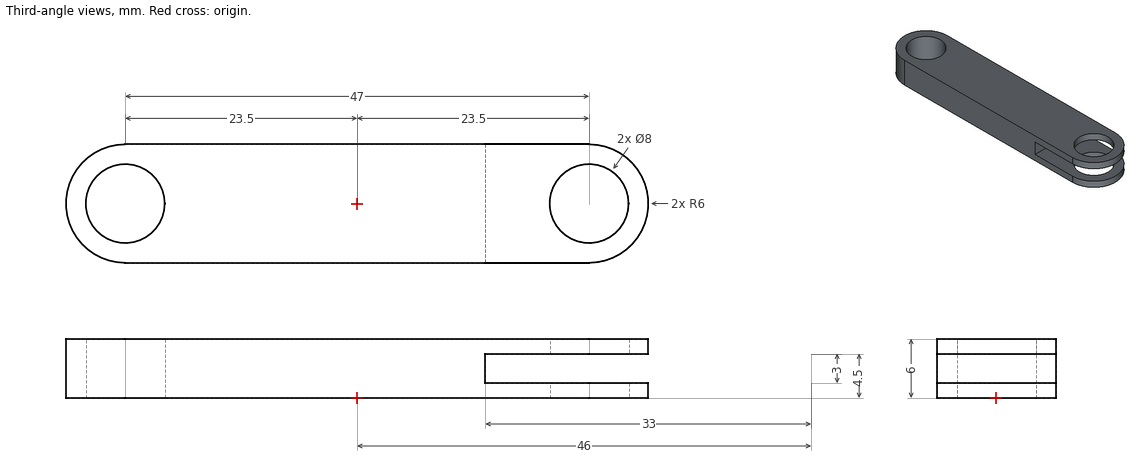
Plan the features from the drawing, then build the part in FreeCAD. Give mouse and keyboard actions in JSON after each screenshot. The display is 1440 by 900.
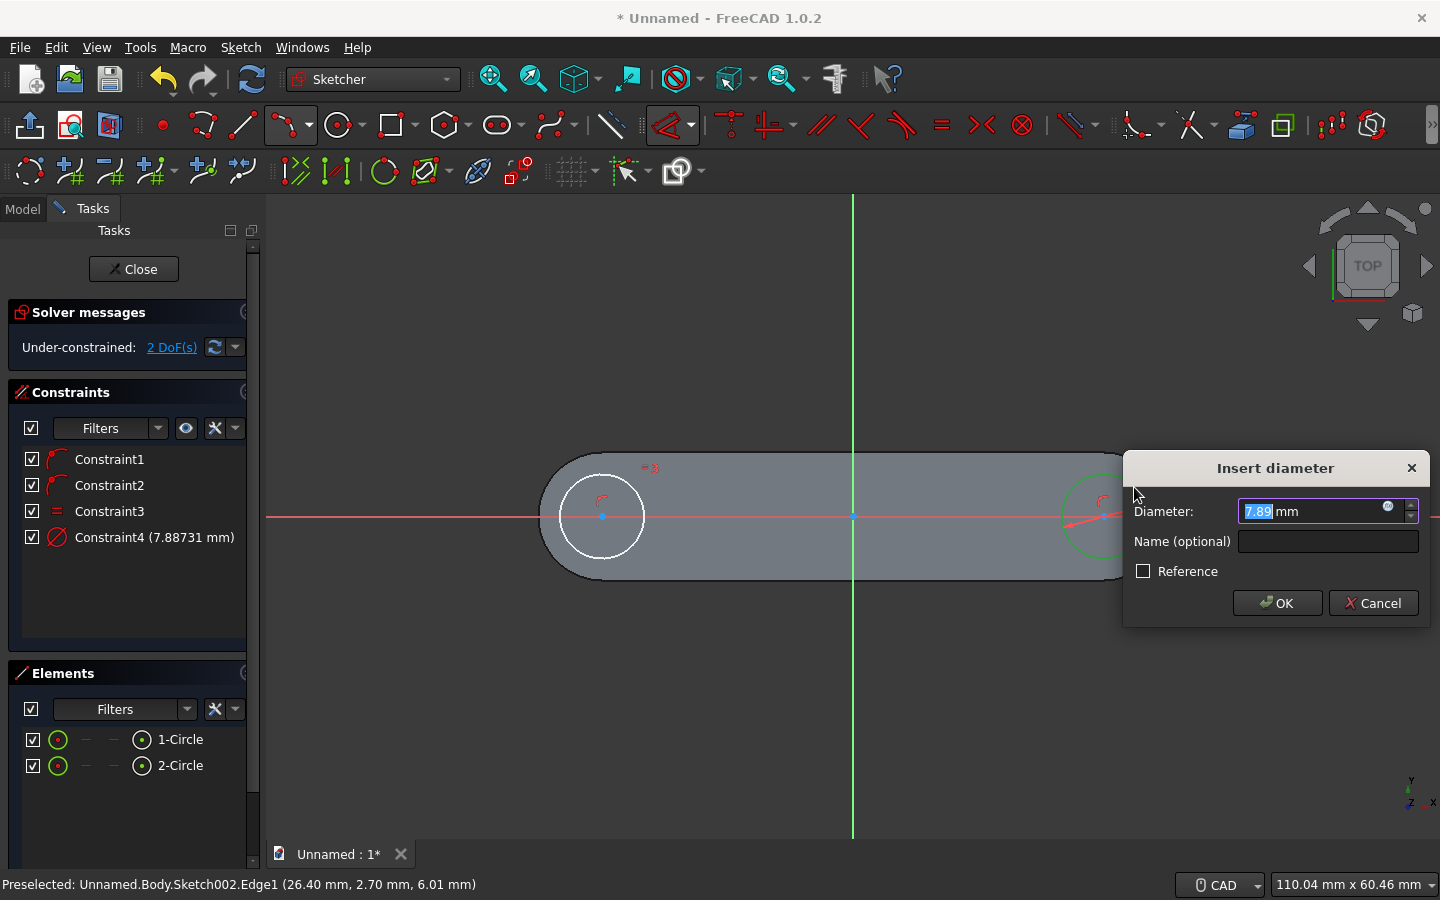
{"action": "type", "text": "8"}
{"action": "key", "text": "Return"}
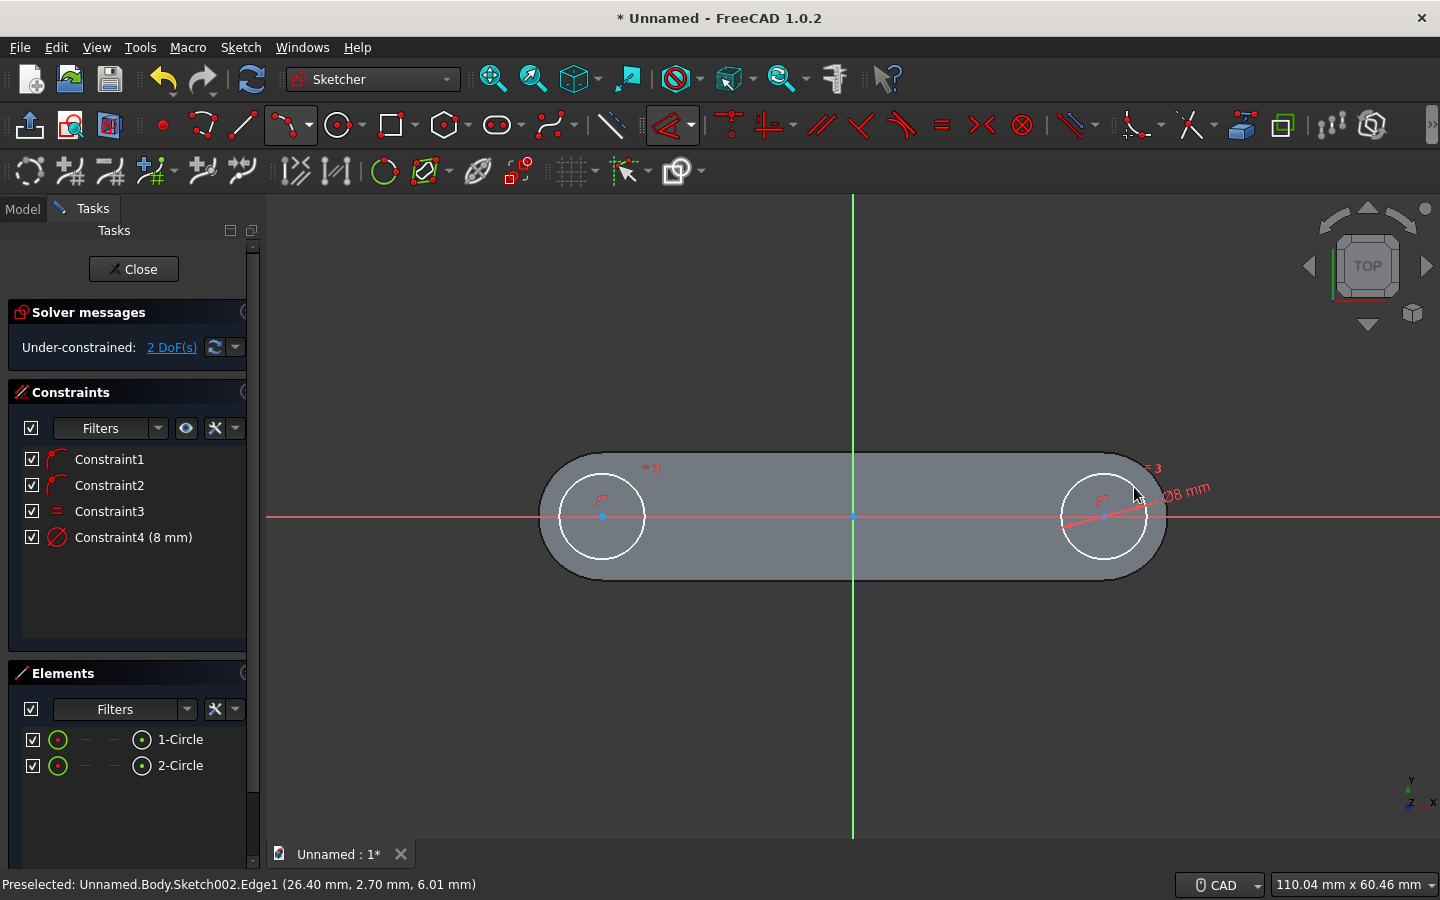
{"action": "left_click", "coordinate": [1104, 516]}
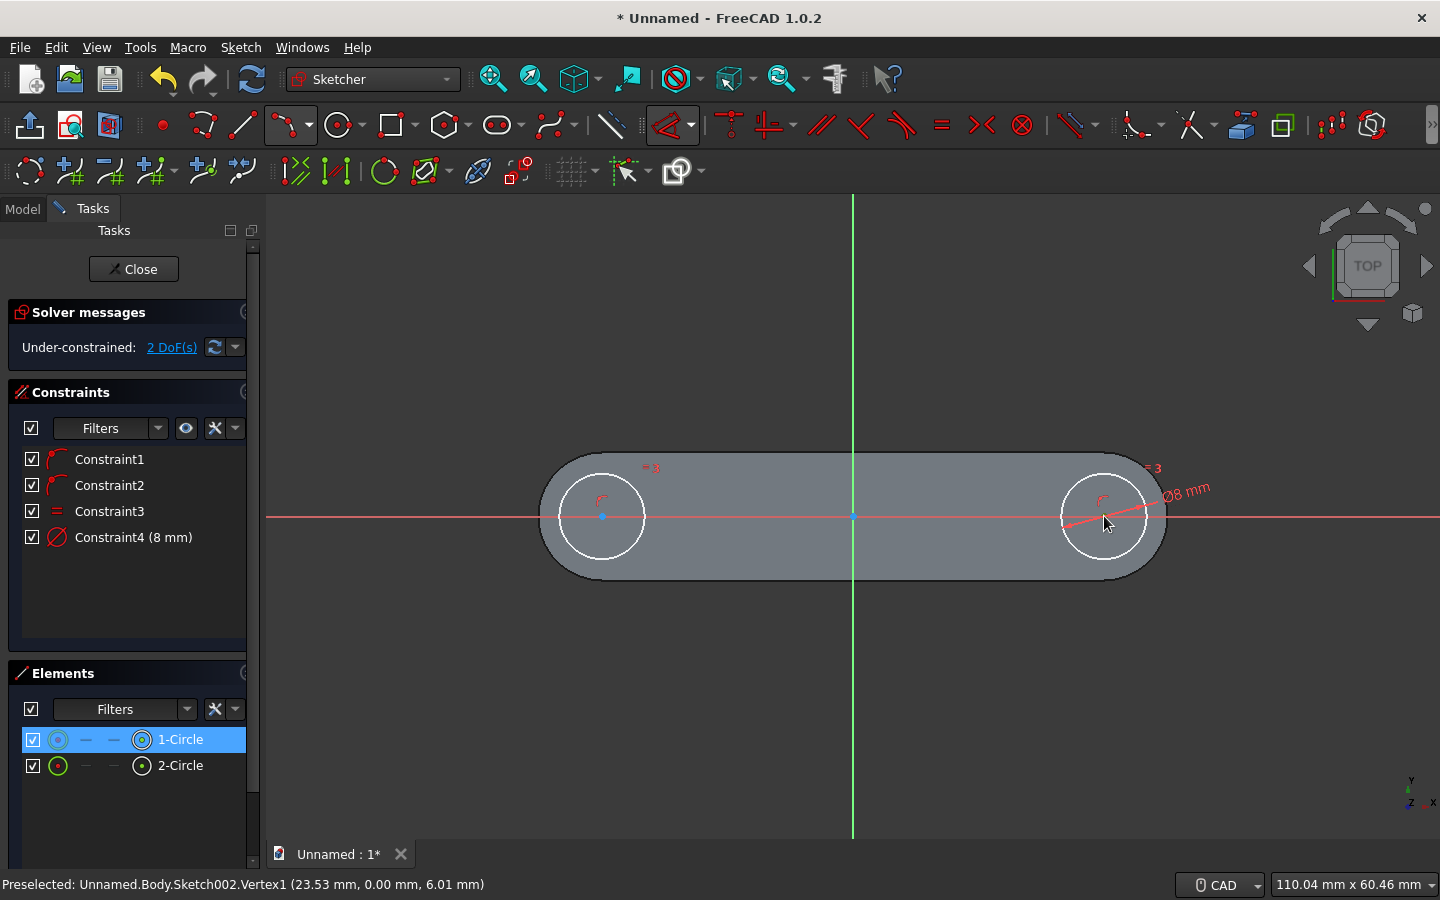
{"action": "left_click", "coordinate": [602, 516]}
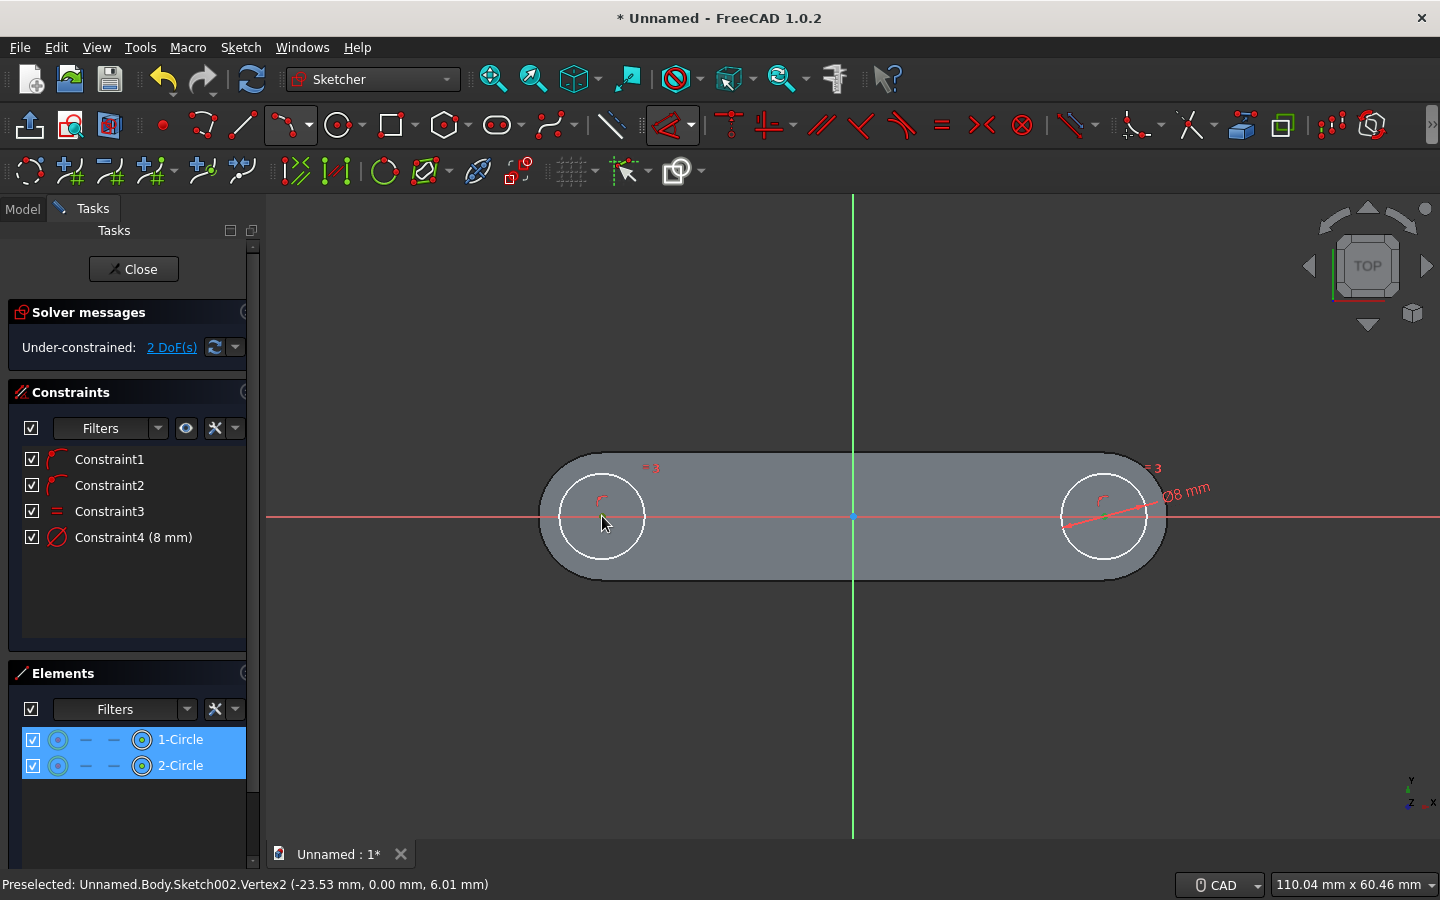
{"action": "key", "text": "l"}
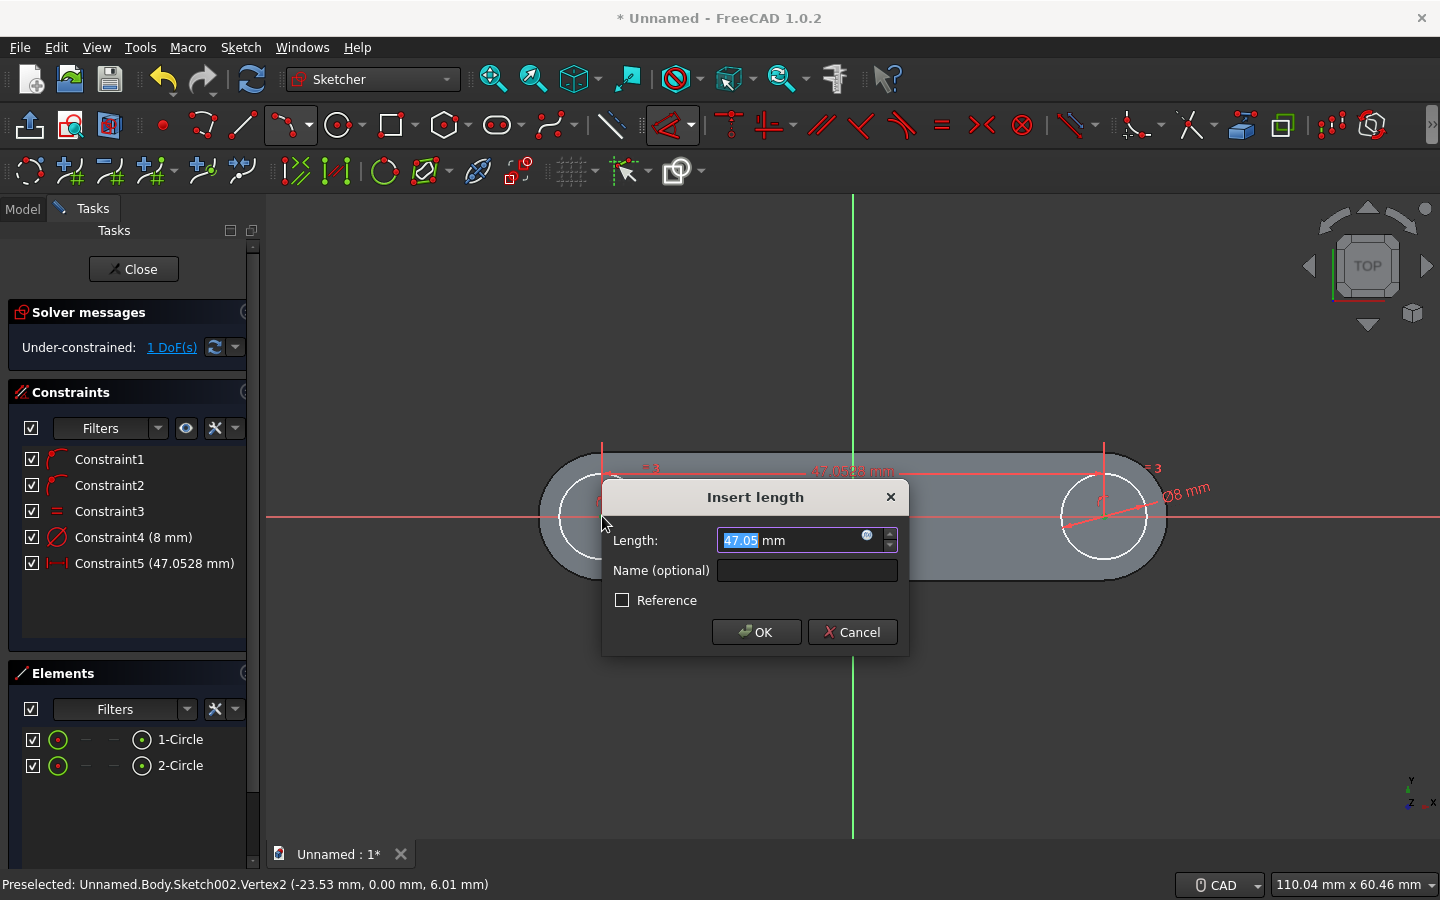
{"action": "type", "text": "47"}
{"action": "key", "text": "Return"}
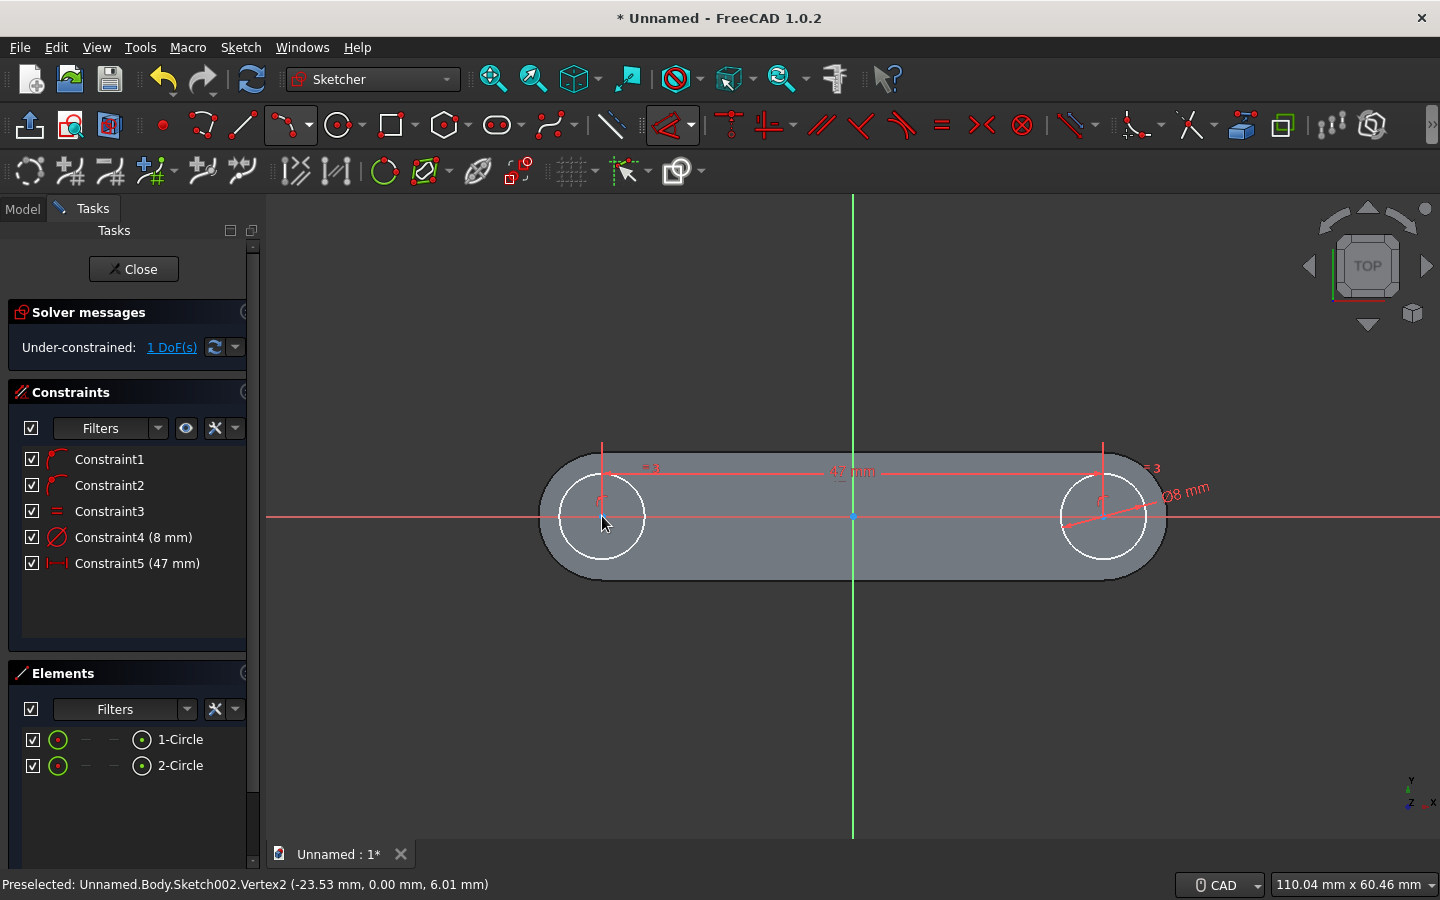
{"action": "left_click", "coordinate": [1103, 516]}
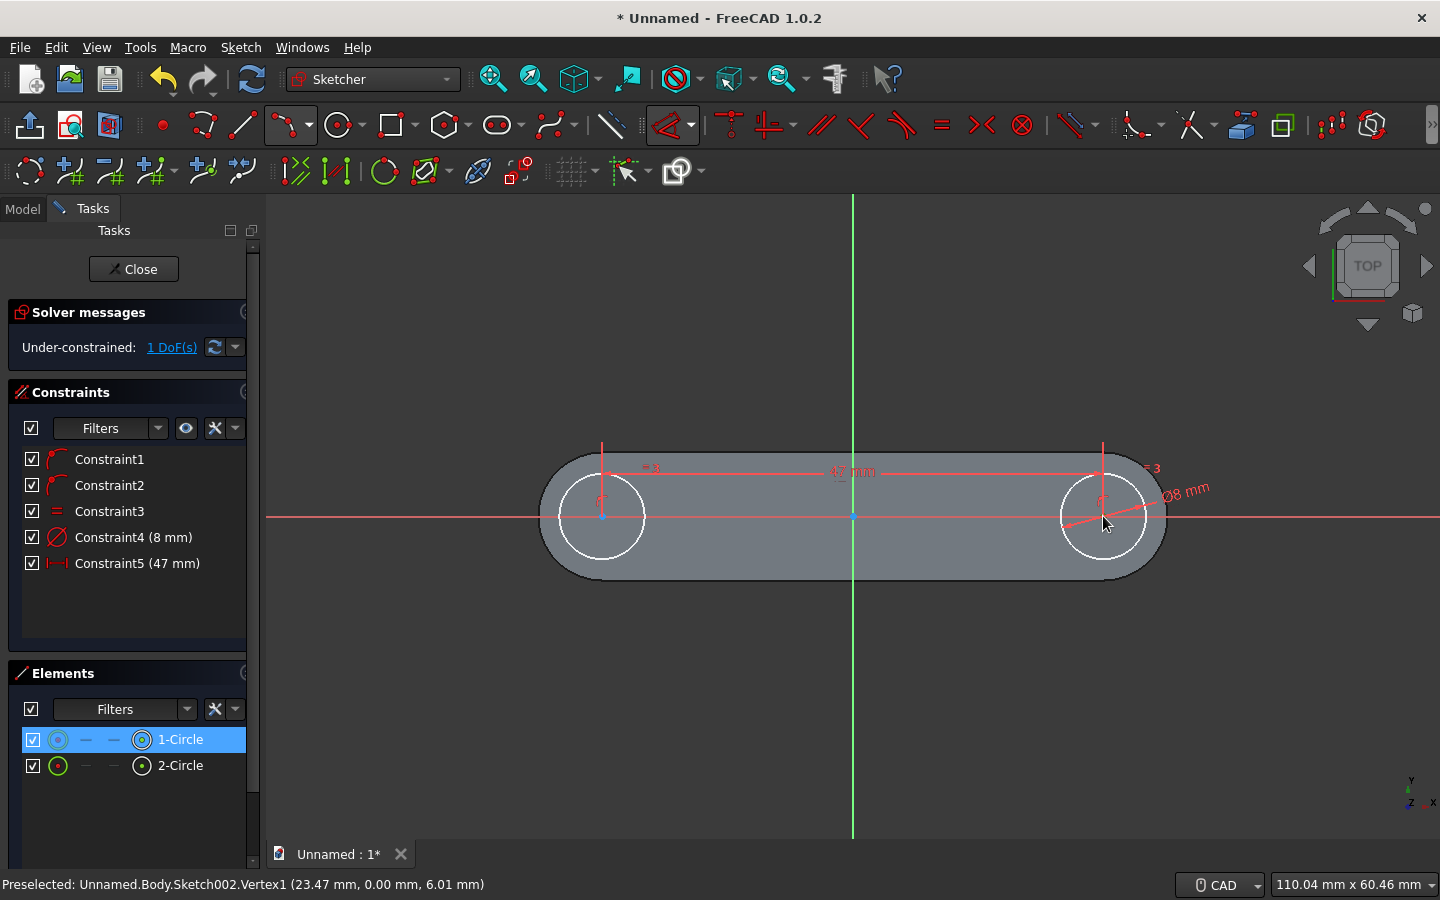
{"action": "key", "text": "l"}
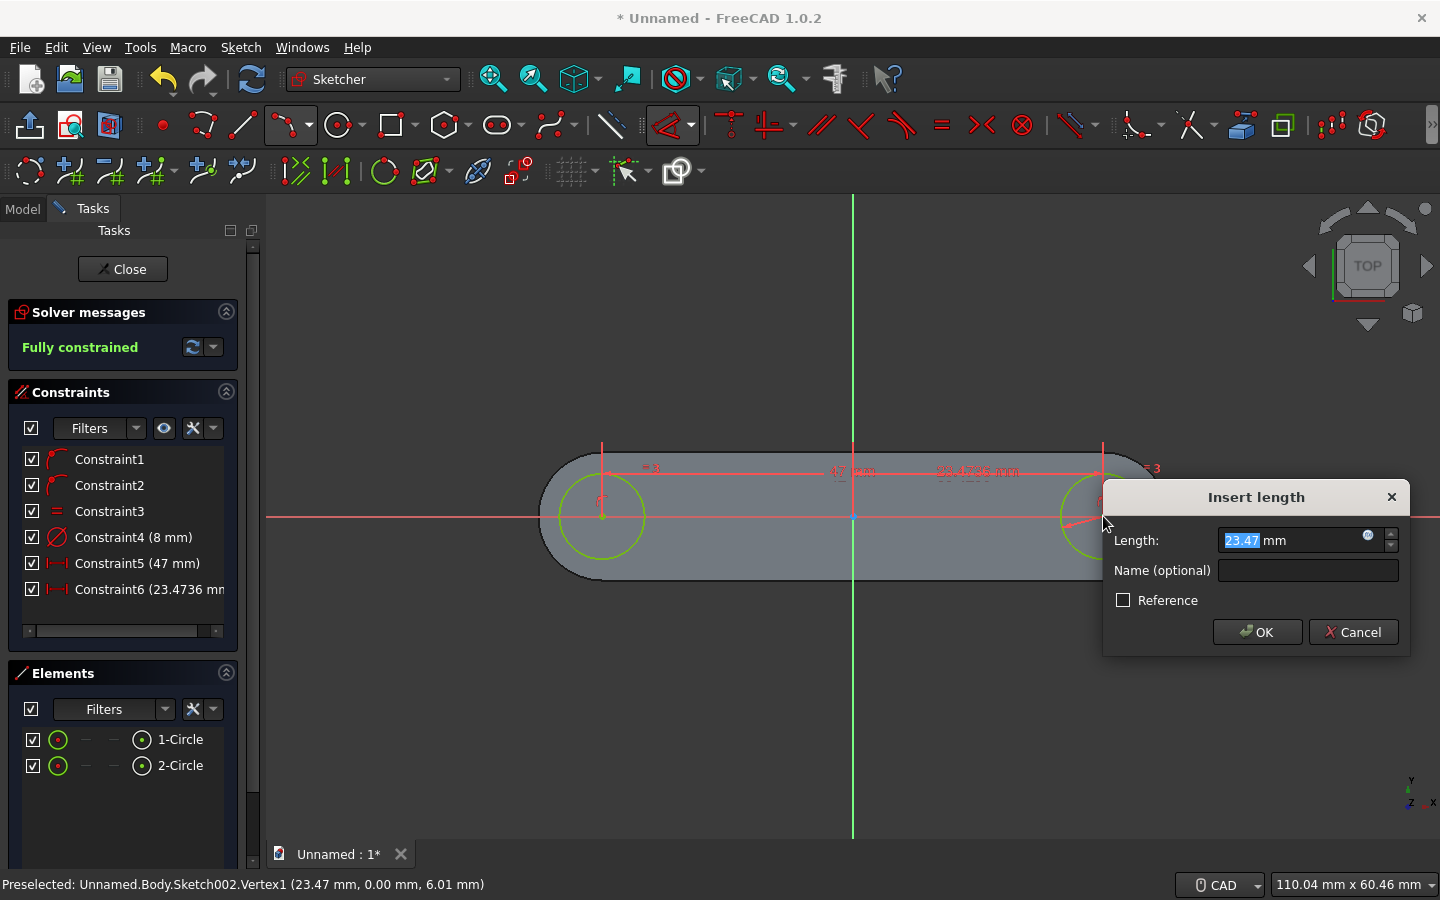
{"action": "type", "text": "23.5"}
{"action": "key", "text": "Return"}